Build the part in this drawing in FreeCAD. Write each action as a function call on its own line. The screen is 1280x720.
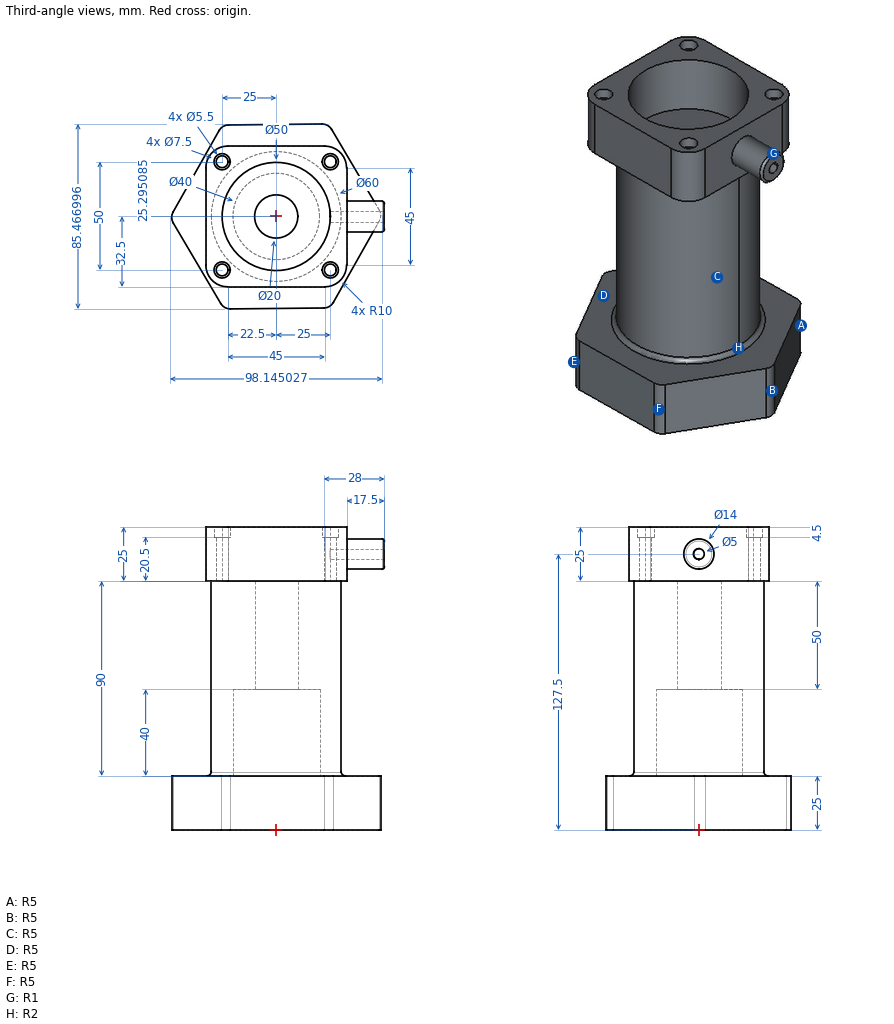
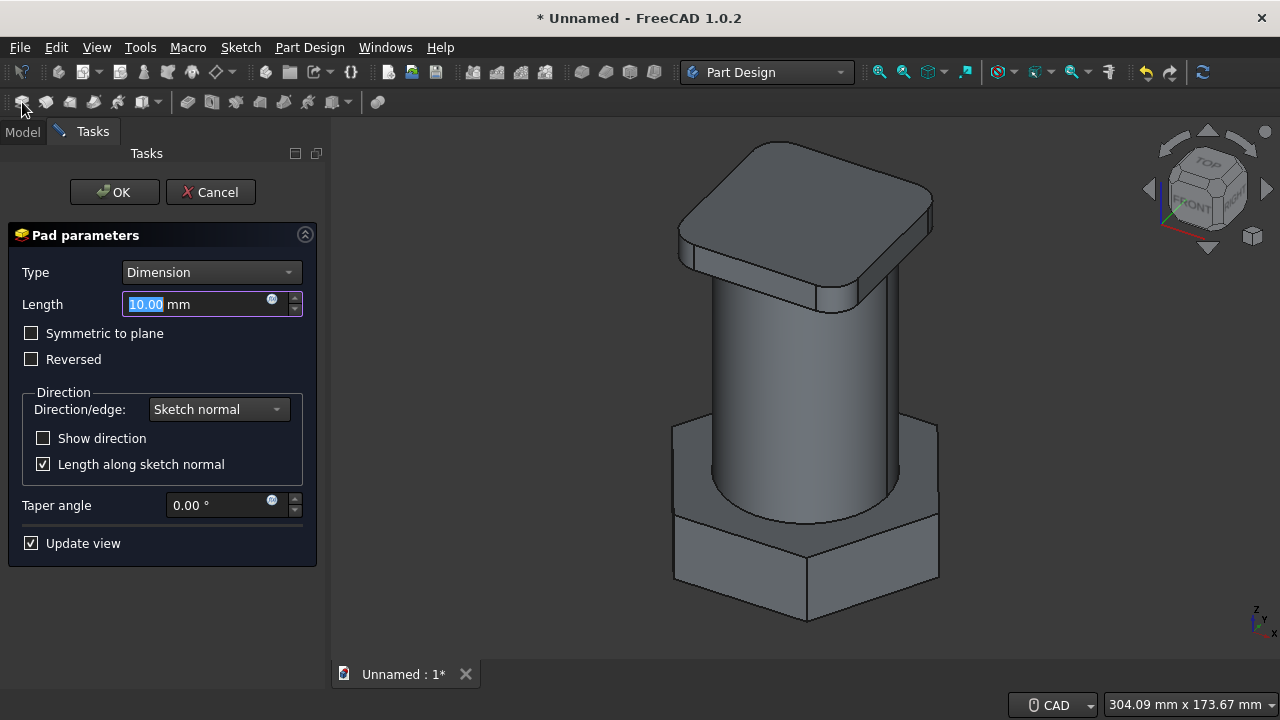
text(25)
key(Tab)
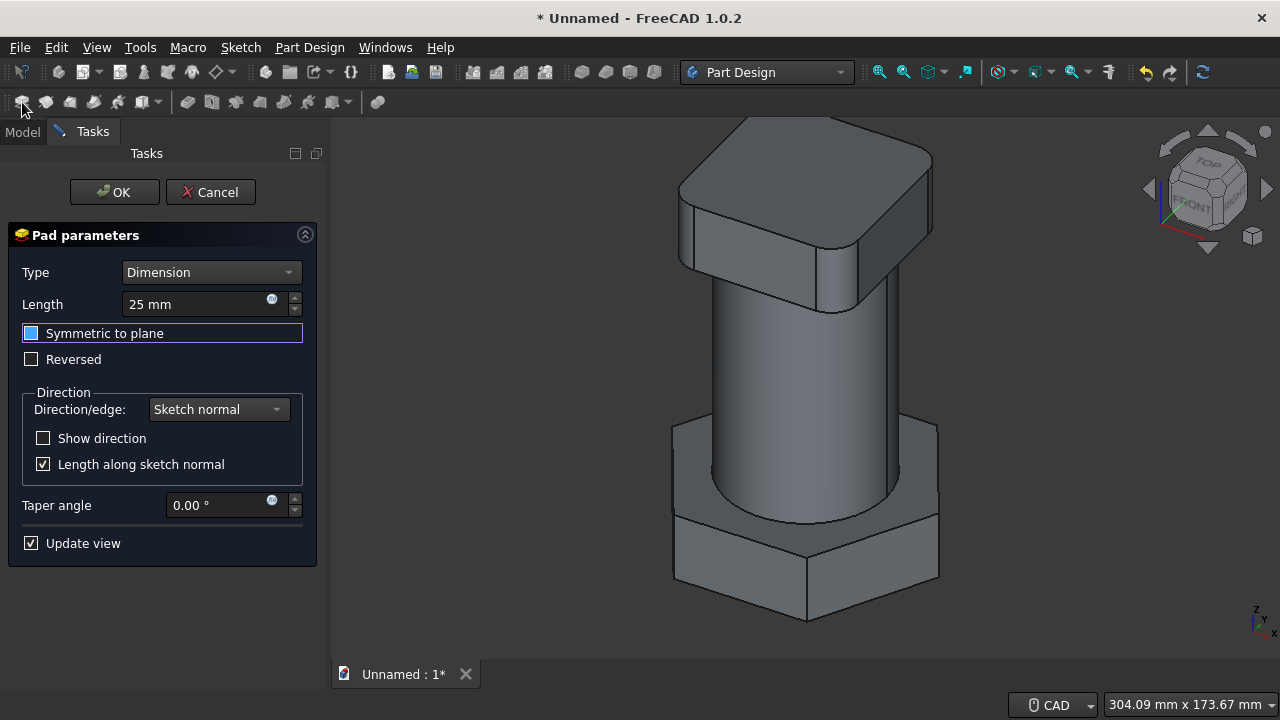
click(115, 192)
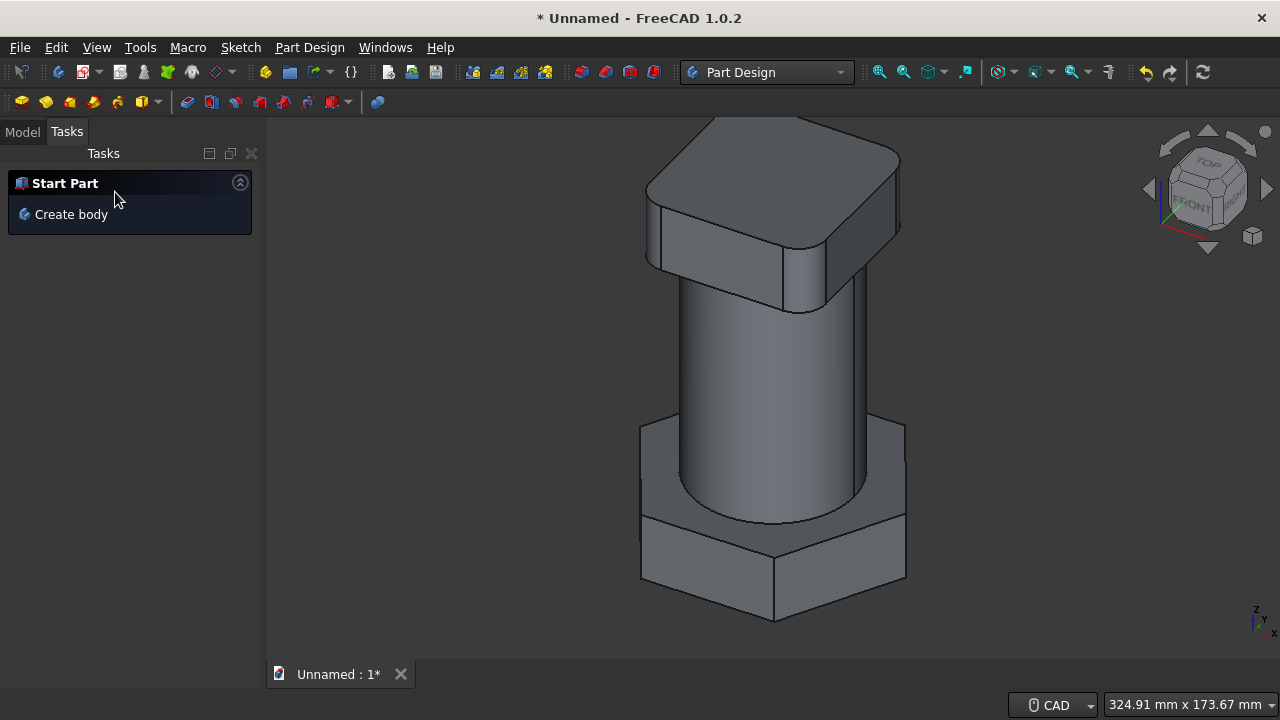
key(v)
key(f)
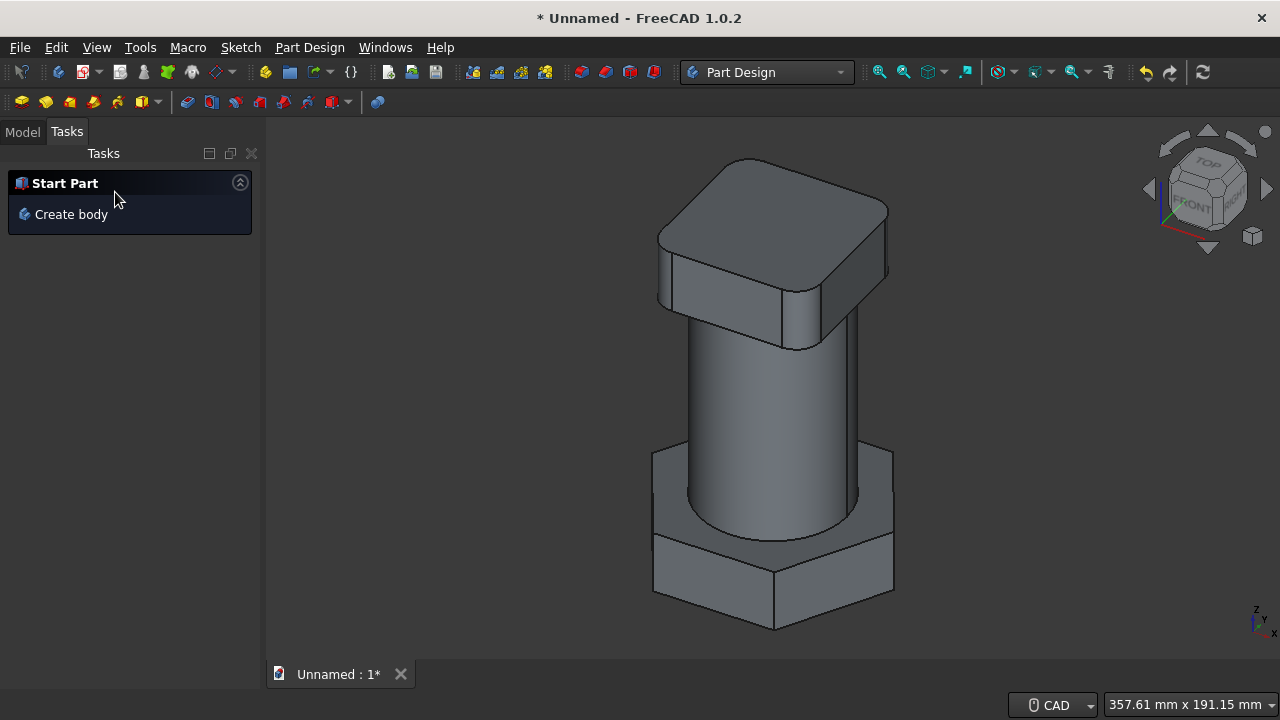
click(773, 224)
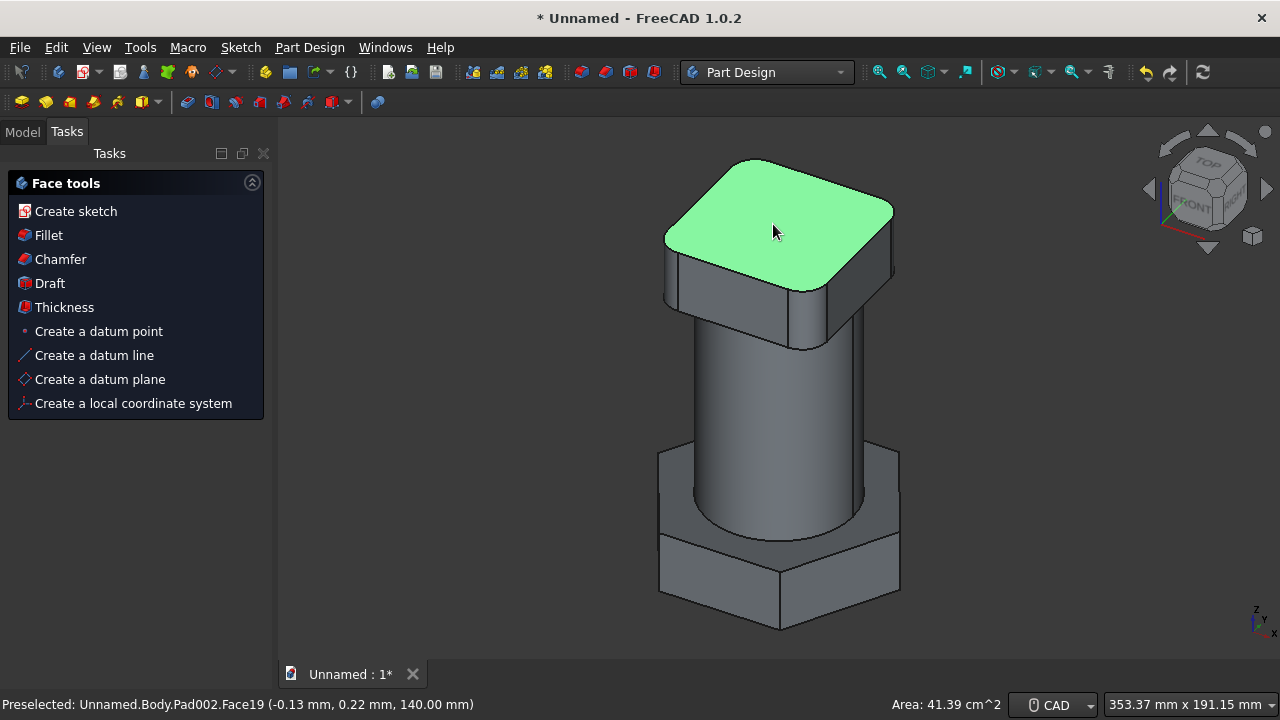
click(84, 72)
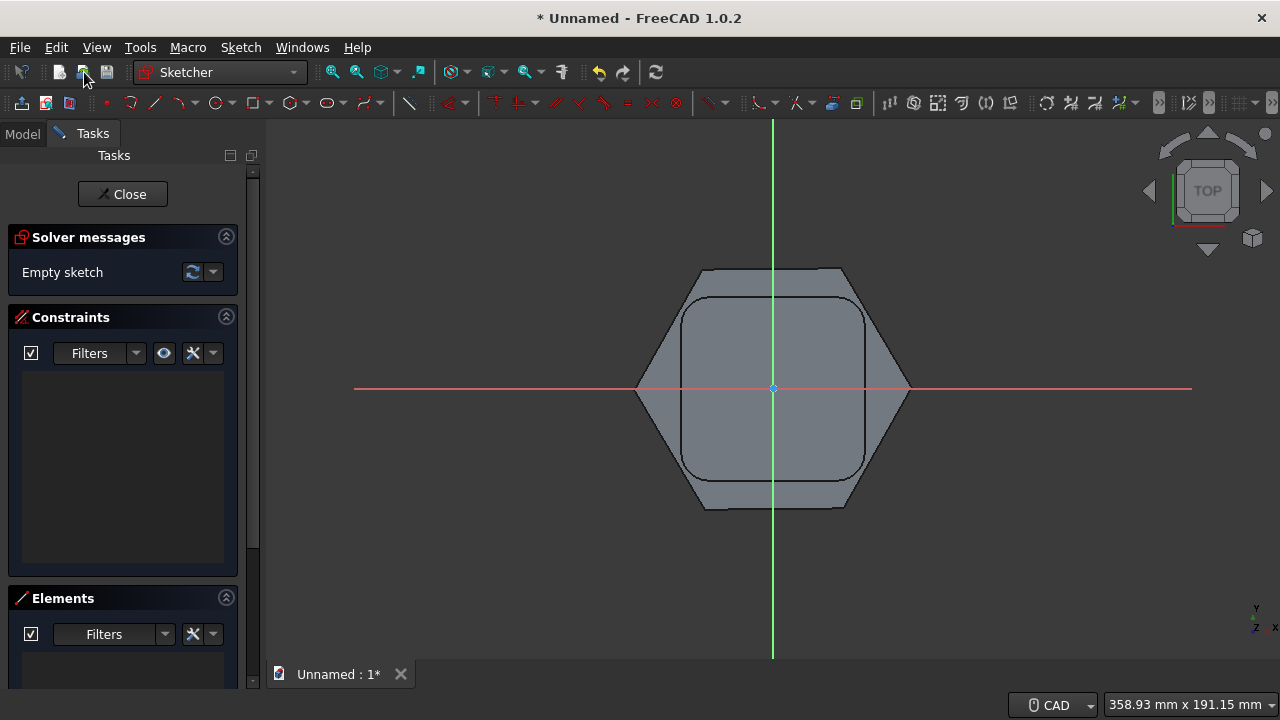
scroll(829, 389, up, 4)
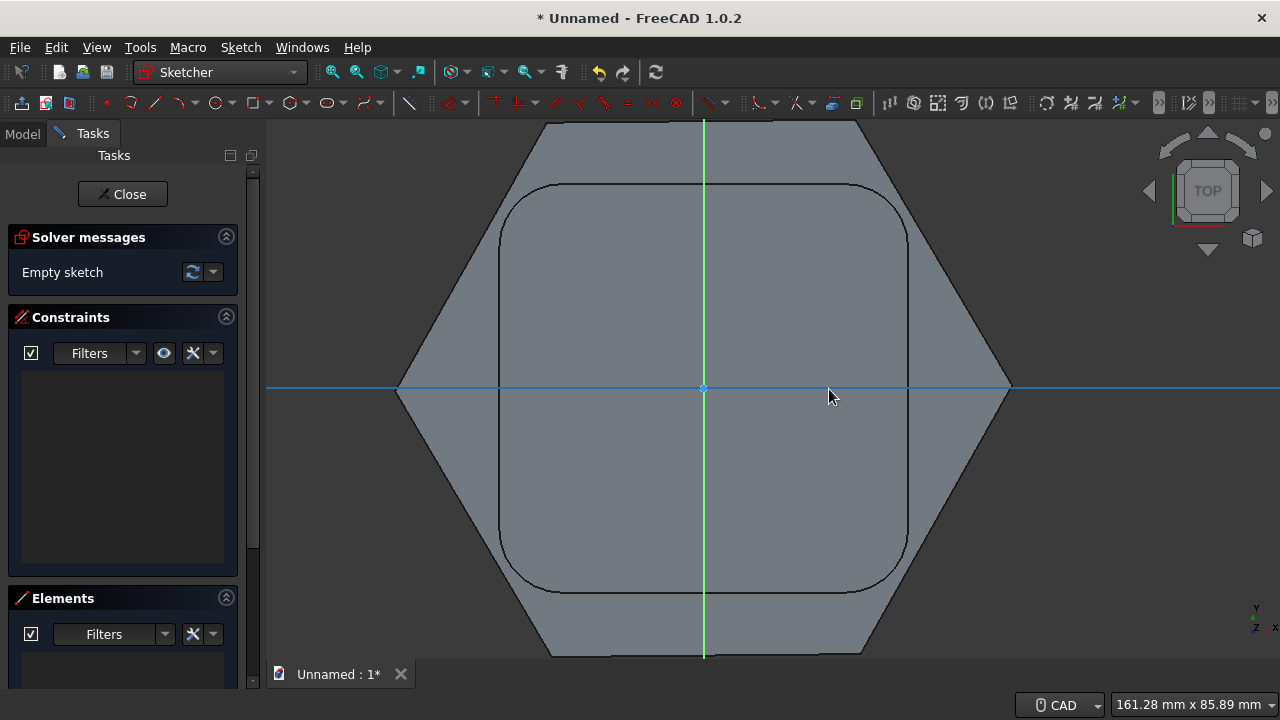
click(216, 104)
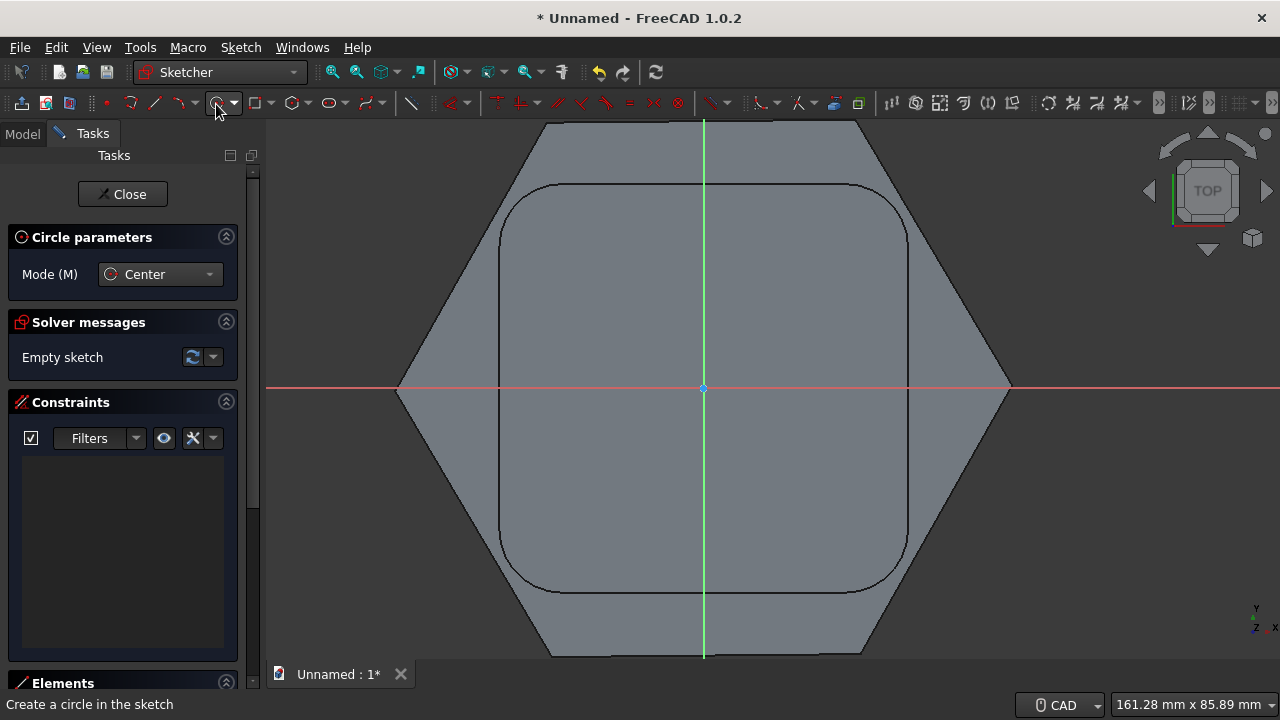
click(704, 388)
click(815, 277)
key(Escape)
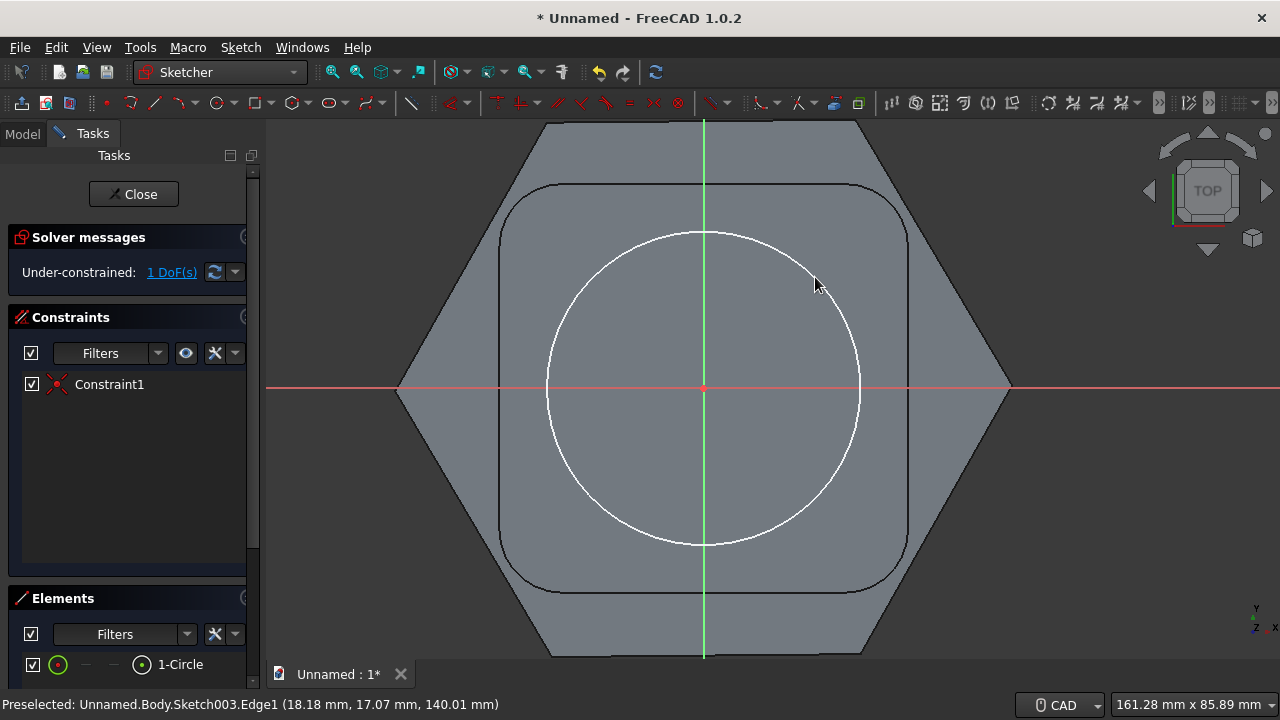
key(d)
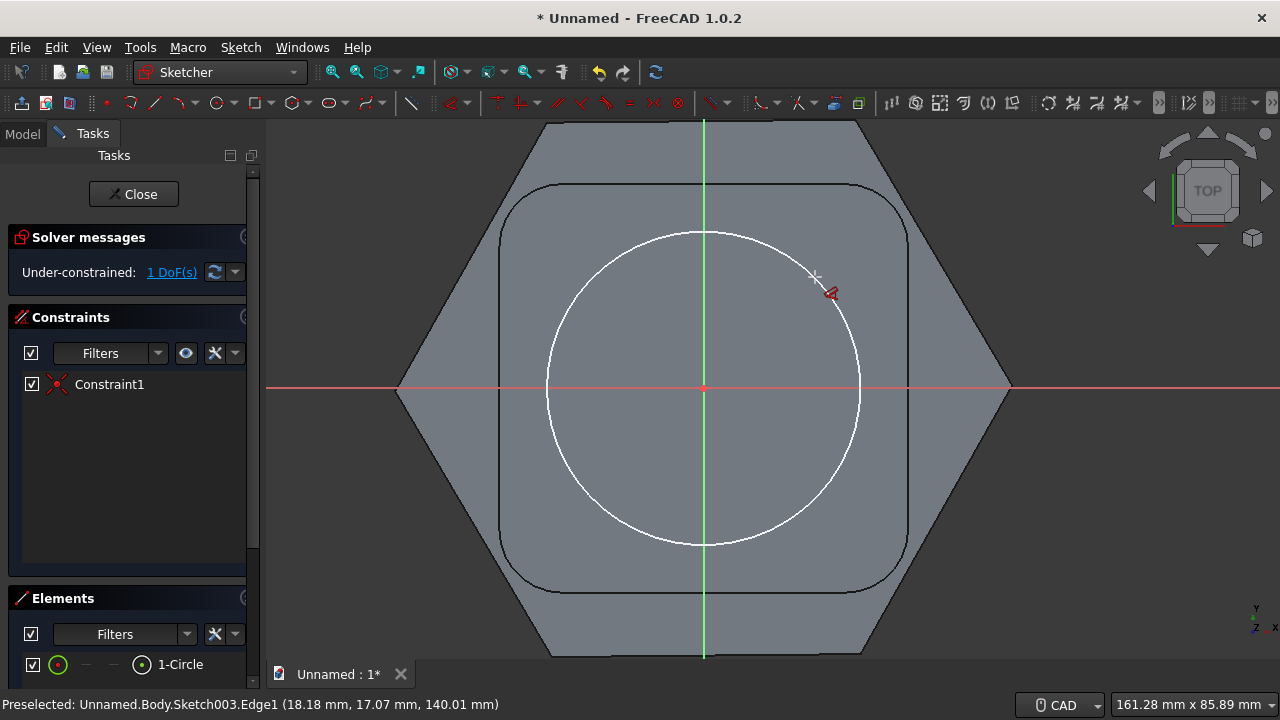
click(814, 277)
click(837, 254)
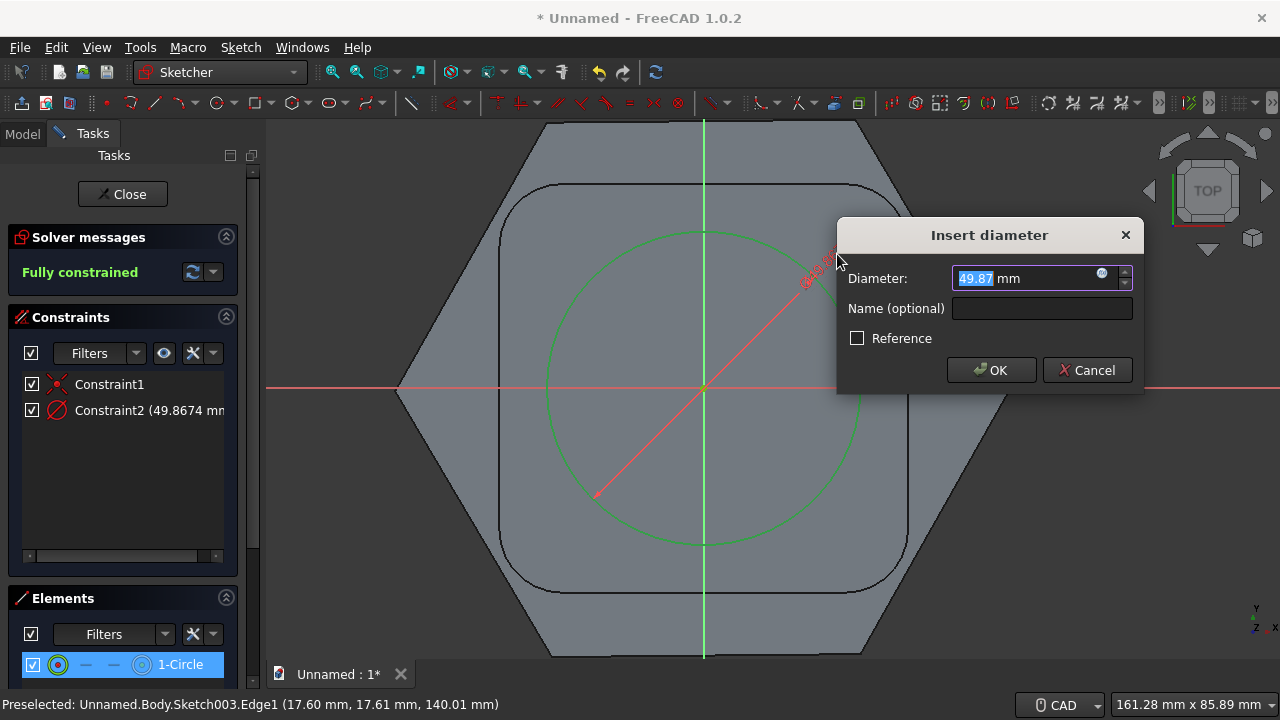
text(50)
key(Return)
key(Escape)